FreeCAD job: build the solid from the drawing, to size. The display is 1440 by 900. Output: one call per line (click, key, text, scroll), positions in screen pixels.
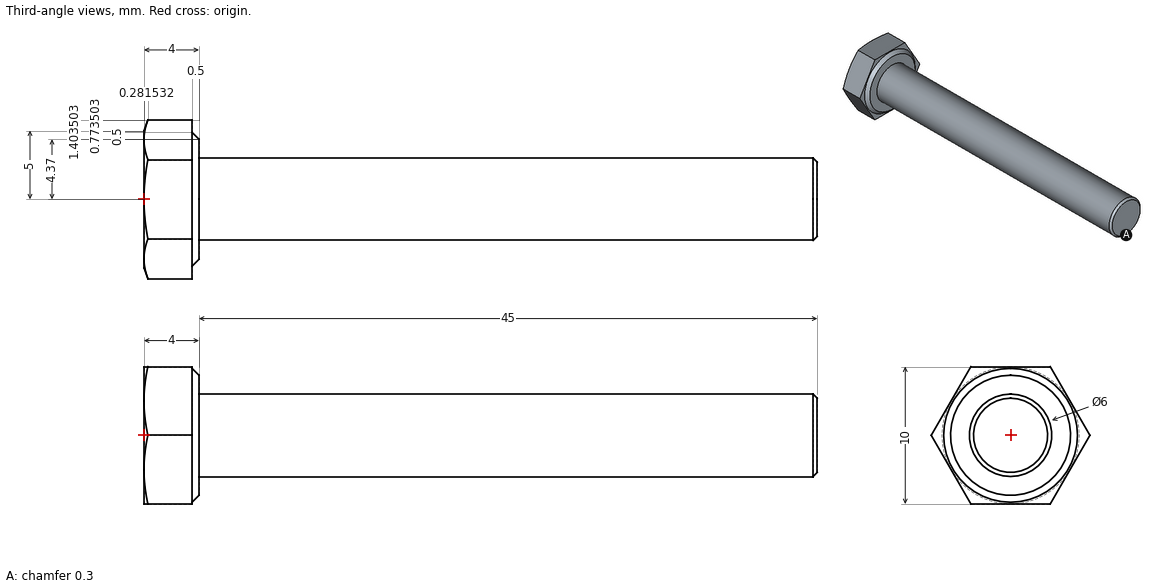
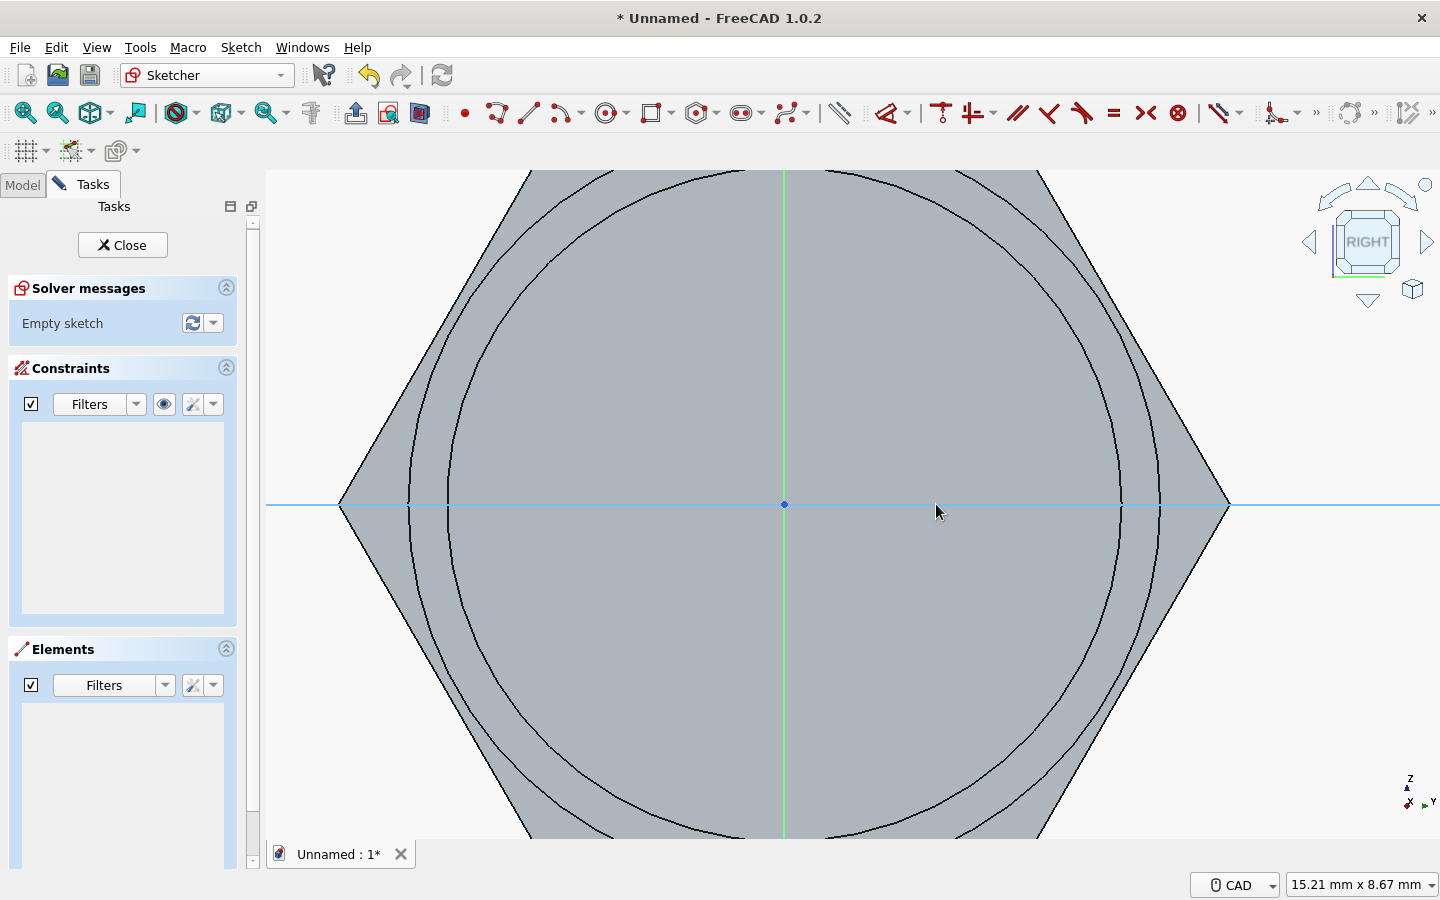
click(606, 114)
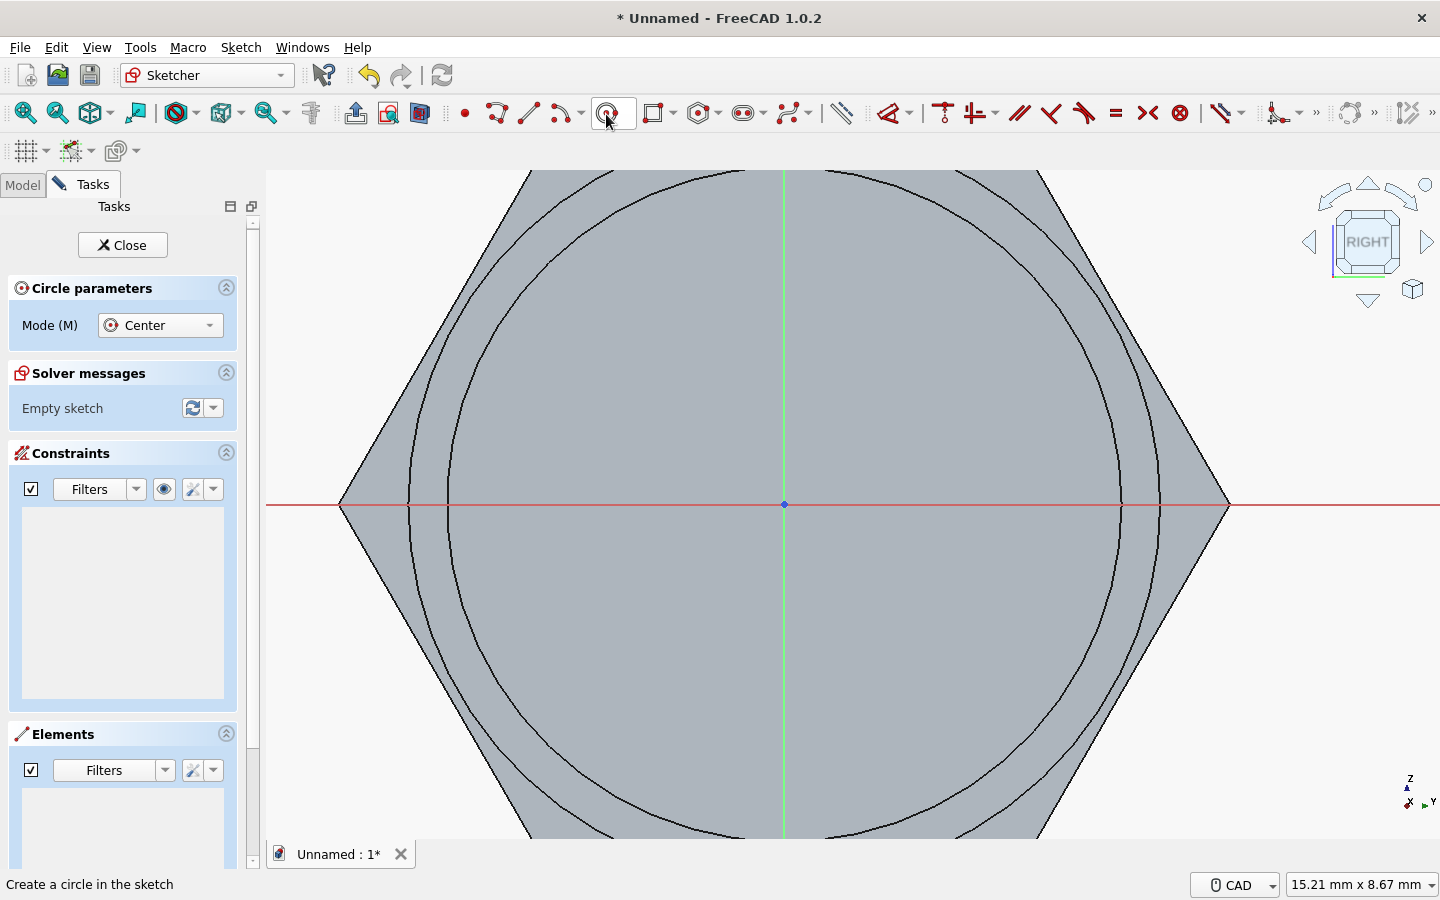
click(784, 504)
click(948, 341)
key(Escape)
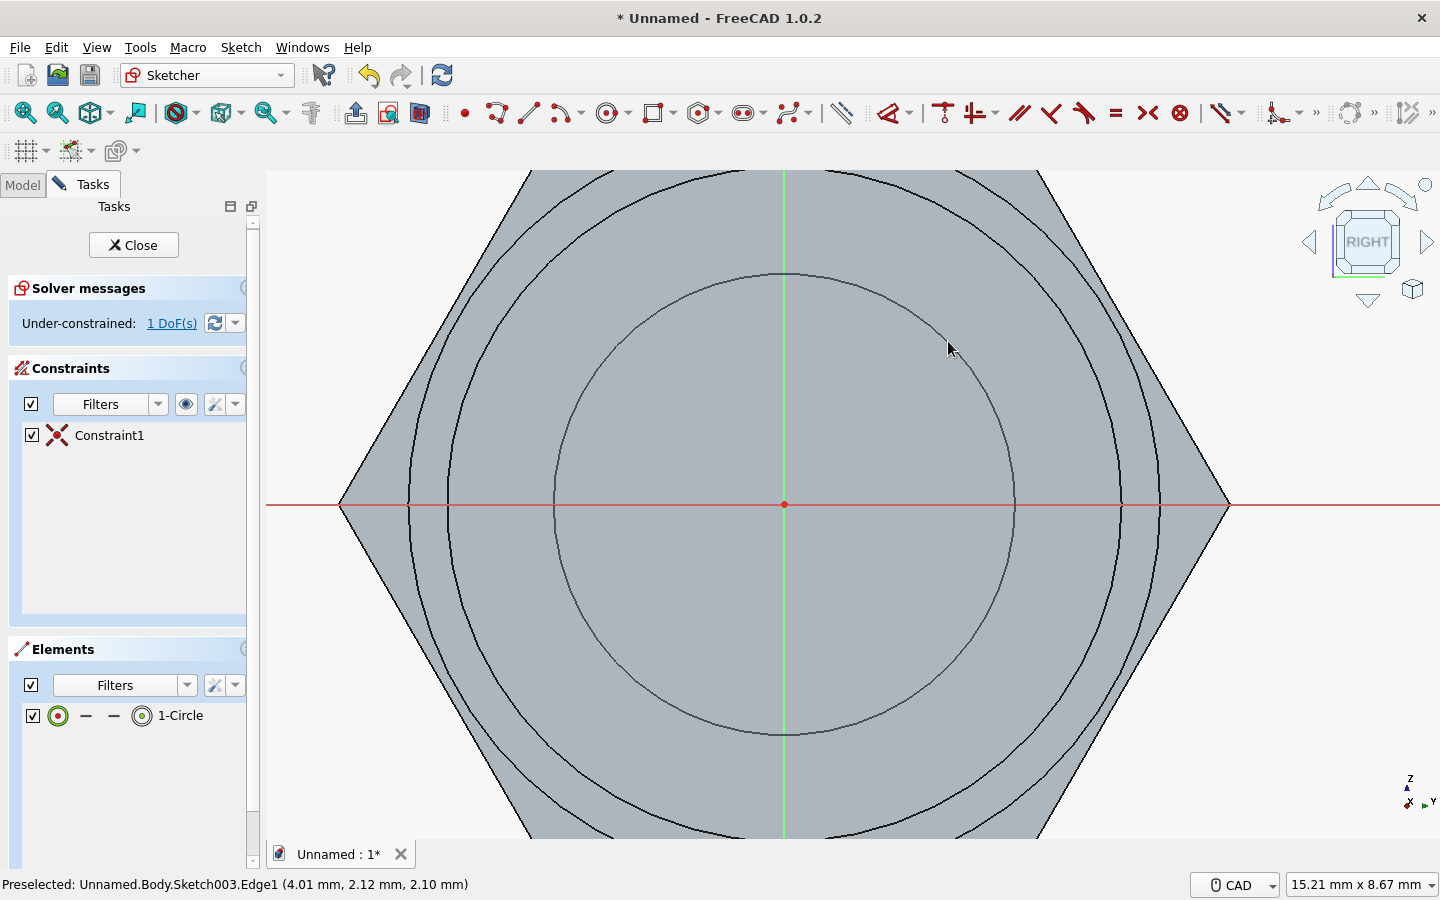
click(888, 114)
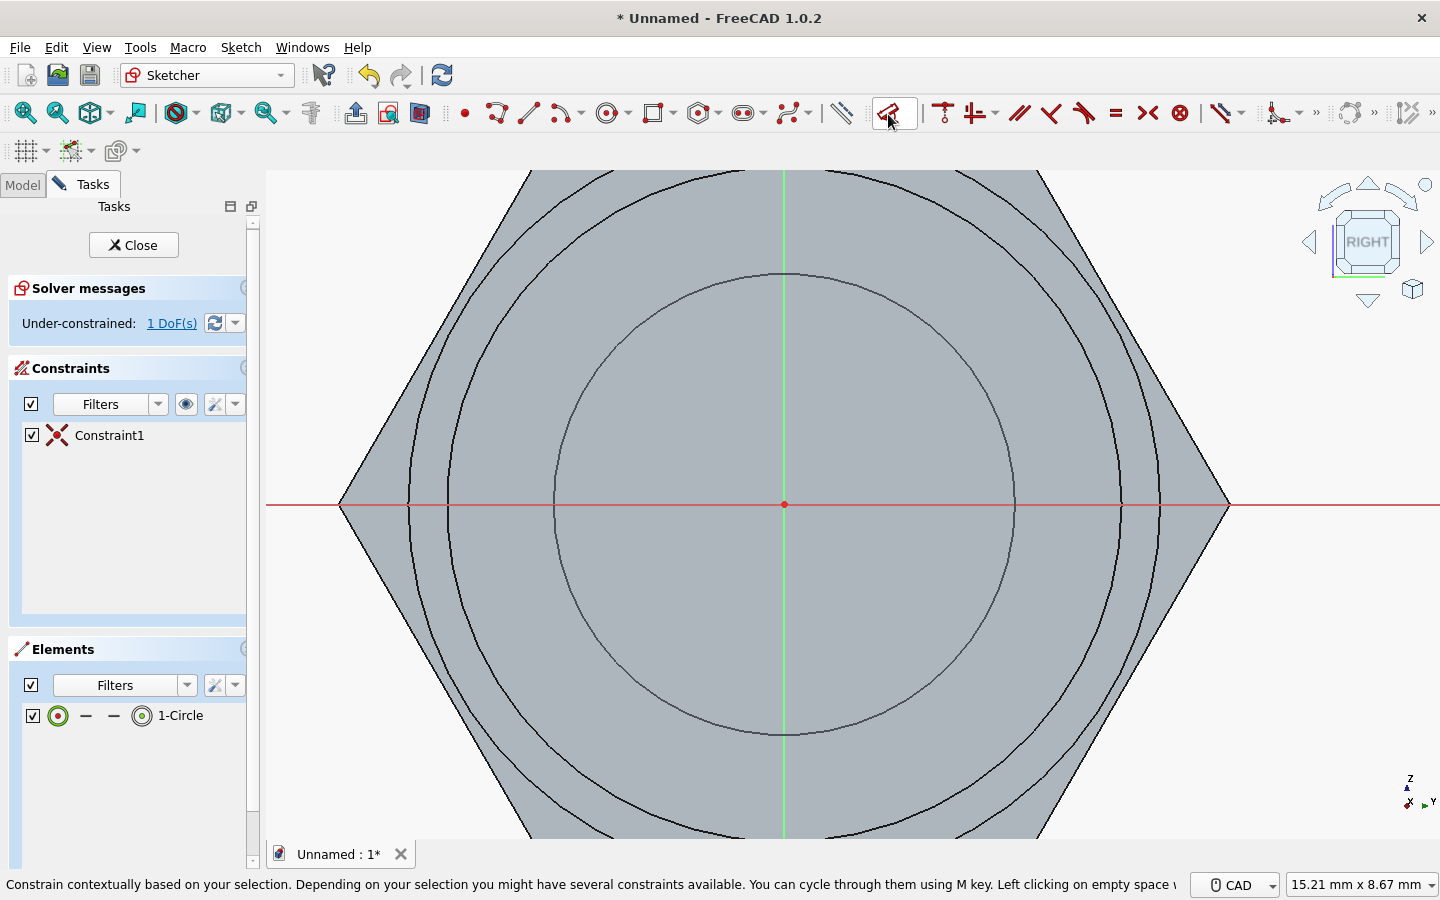
click(947, 341)
click(970, 318)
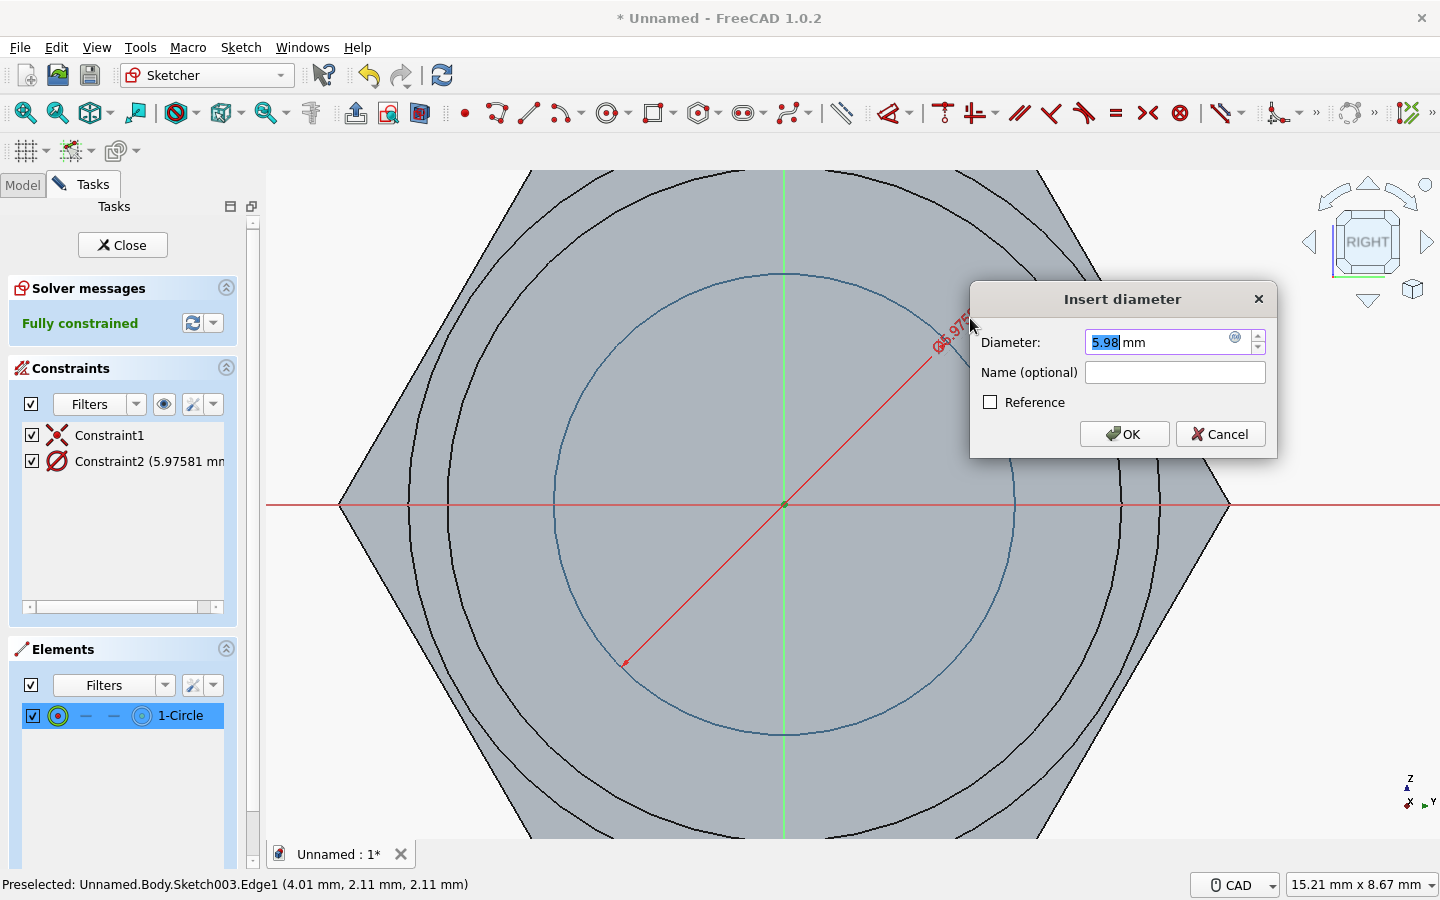
text(6)
key(Return)
key(Escape)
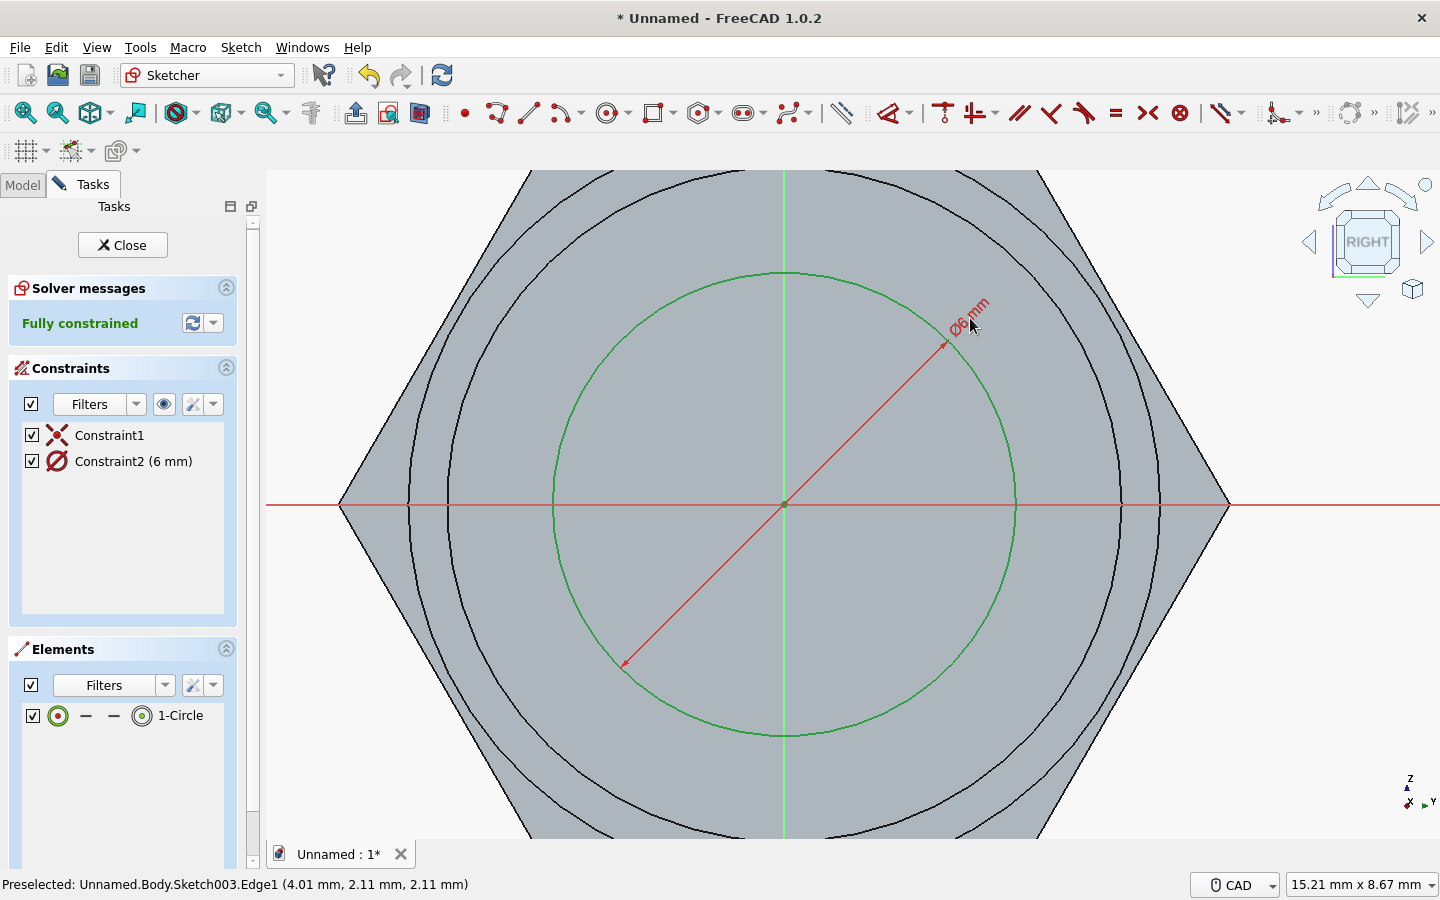
click(123, 245)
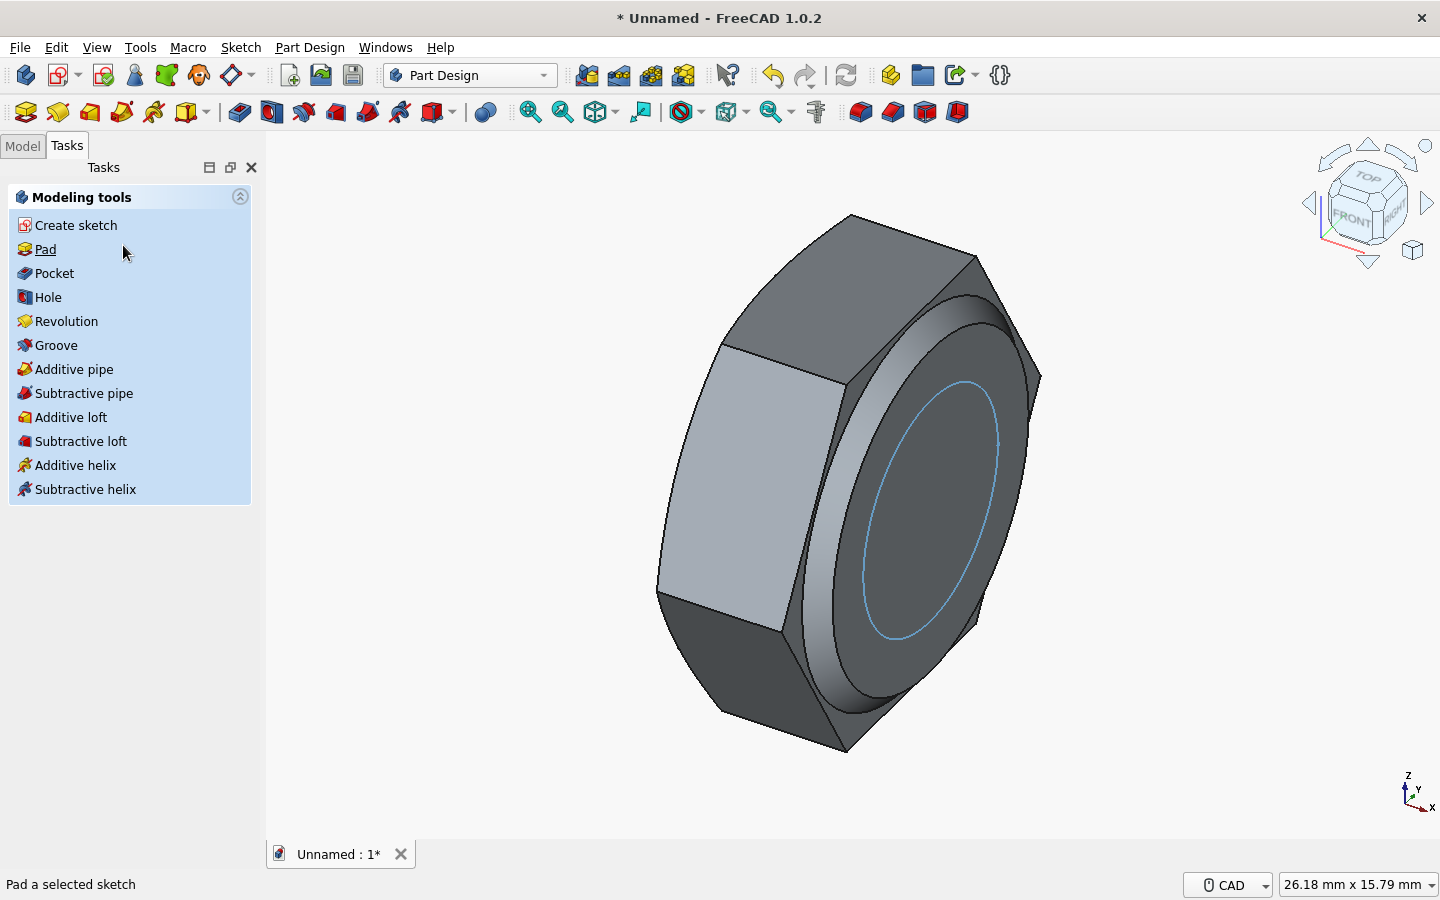
click(26, 112)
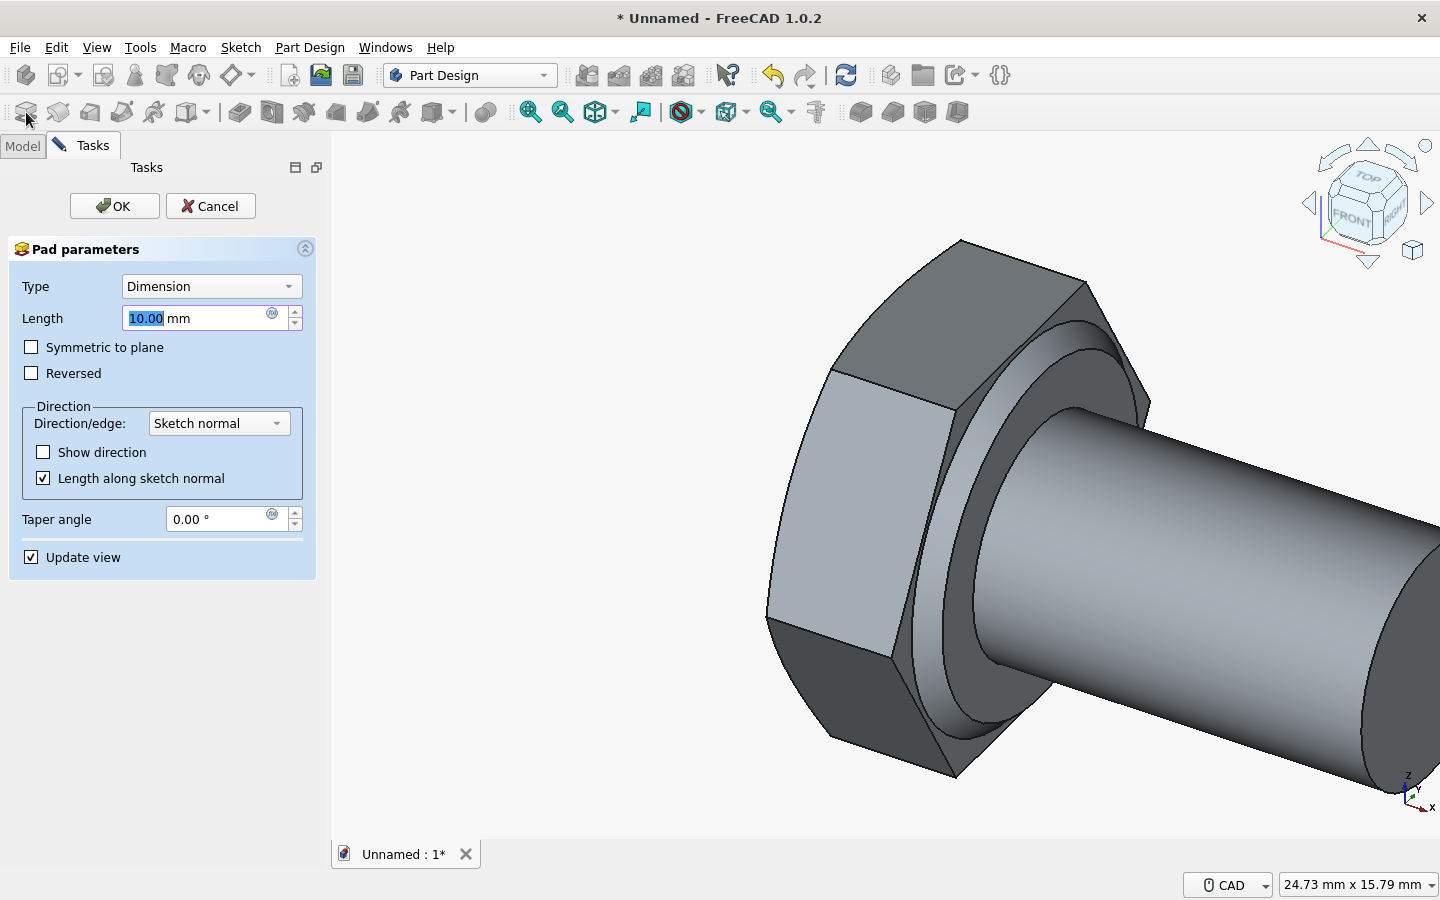
text(45)
key(Tab)